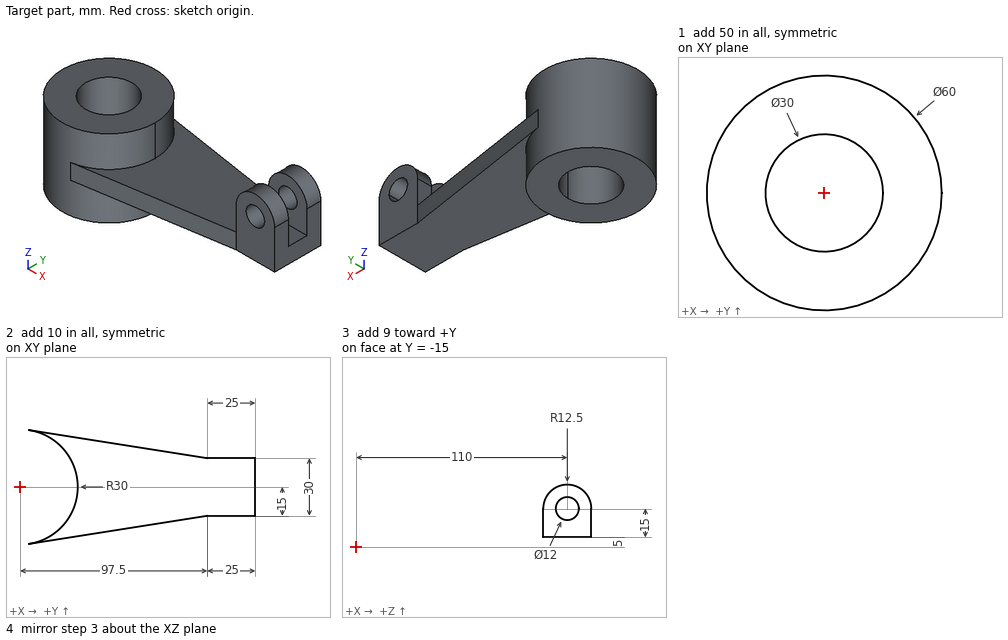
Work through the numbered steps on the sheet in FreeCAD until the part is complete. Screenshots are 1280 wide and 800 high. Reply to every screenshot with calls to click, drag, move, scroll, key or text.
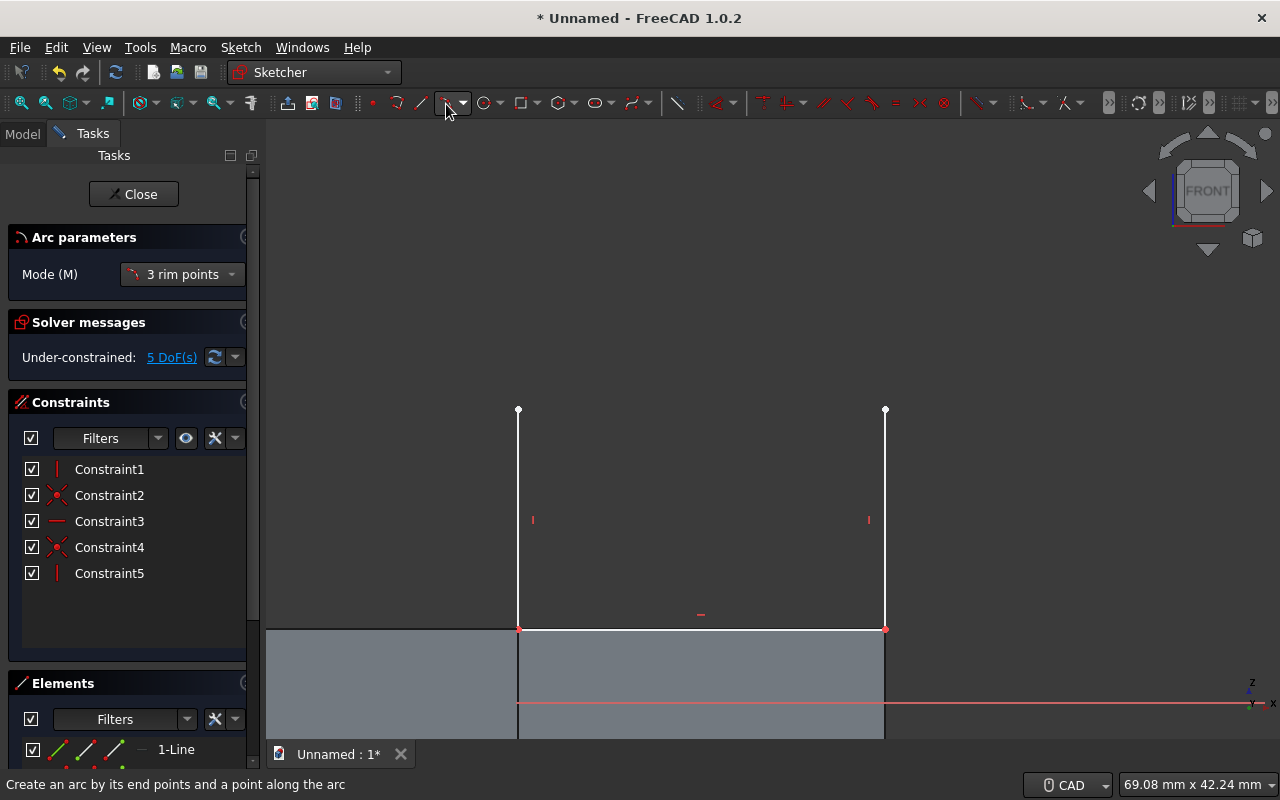
click(885, 410)
click(518, 410)
click(701, 226)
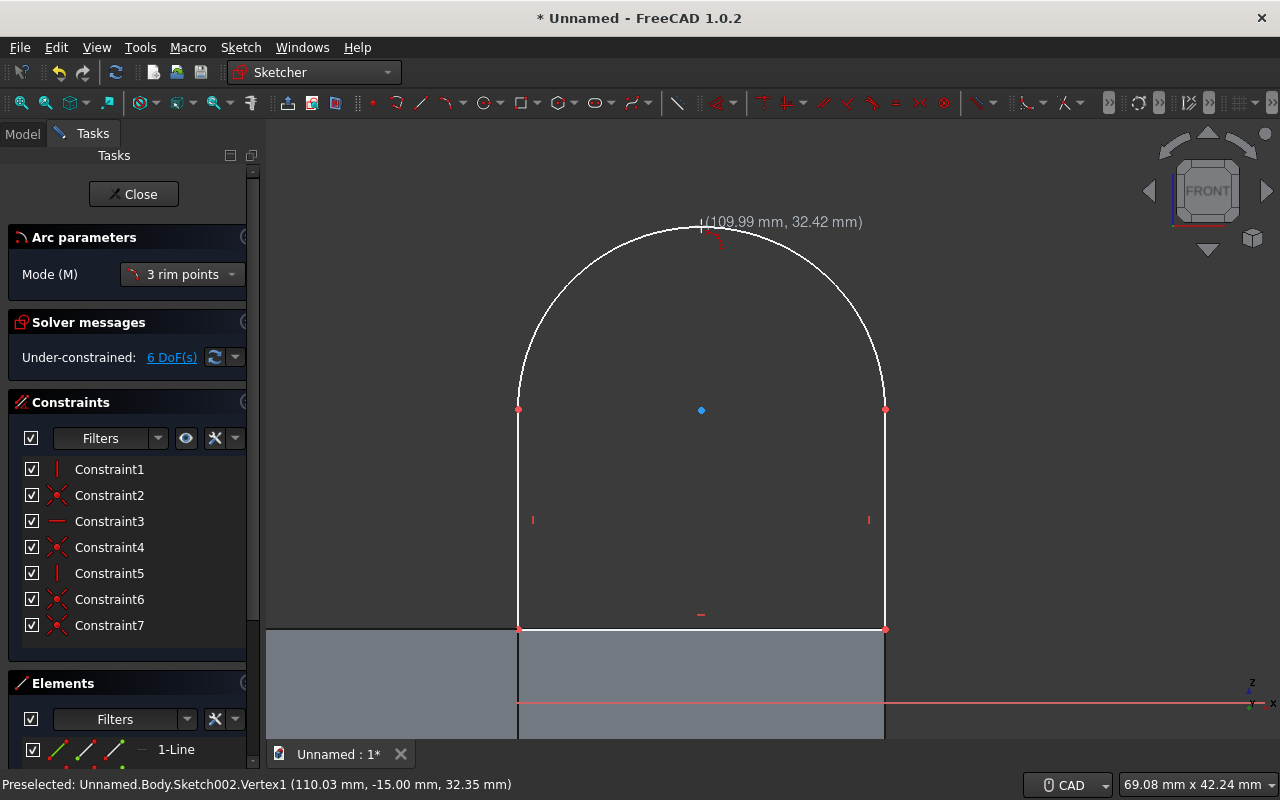
click(484, 104)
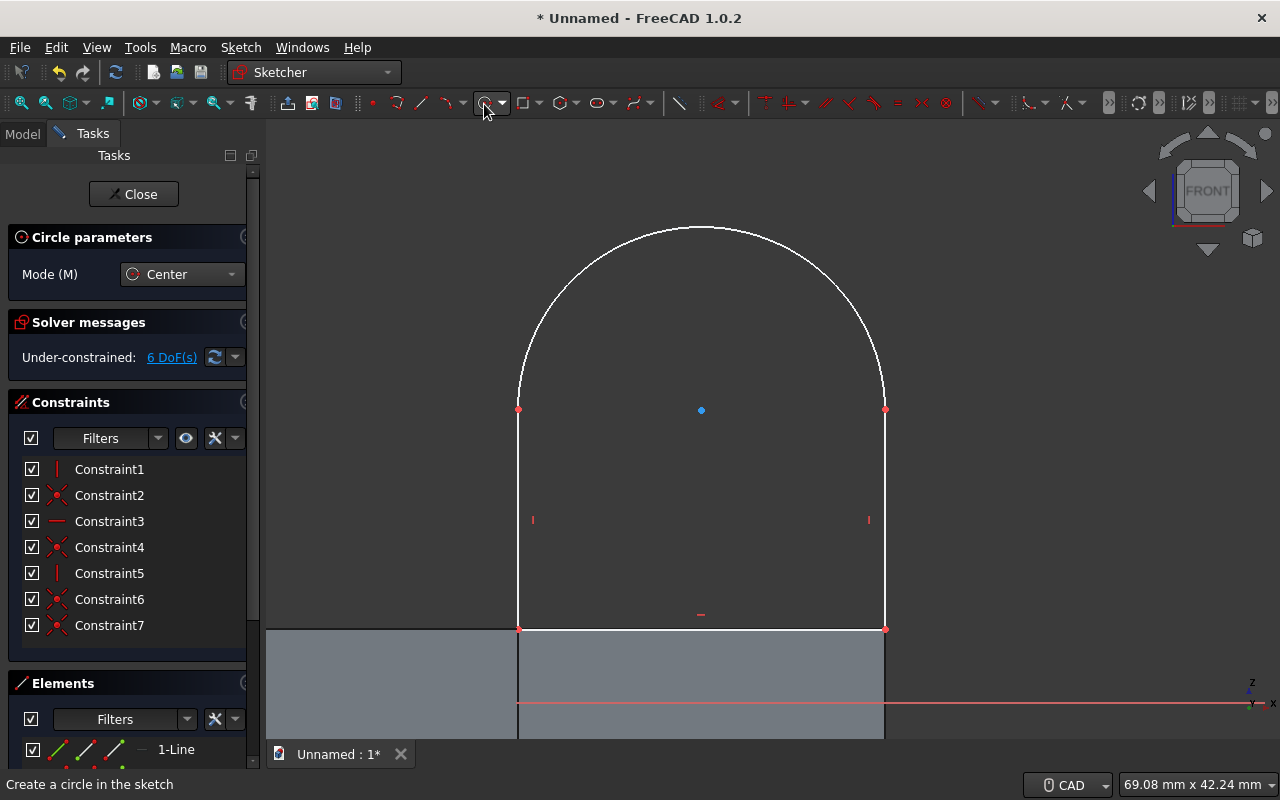
click(701, 409)
click(763, 347)
key(Escape)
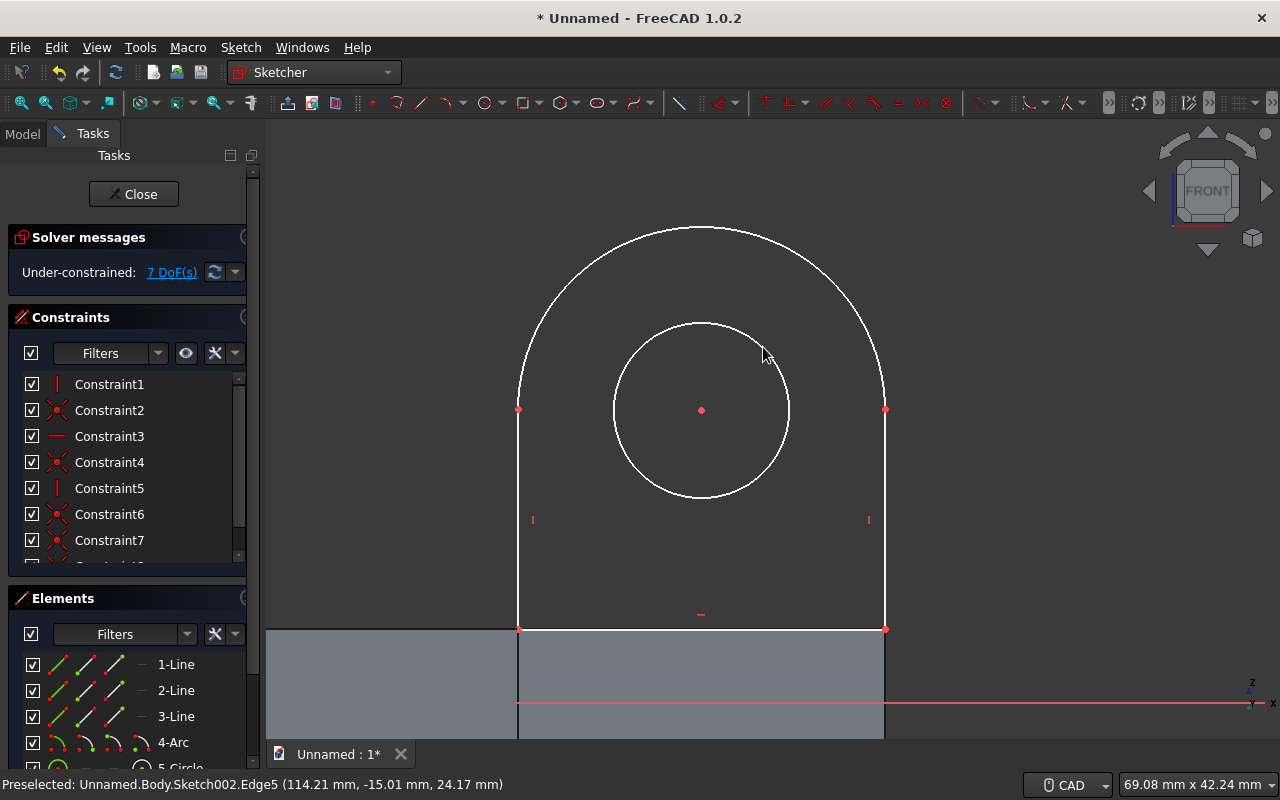
click(518, 476)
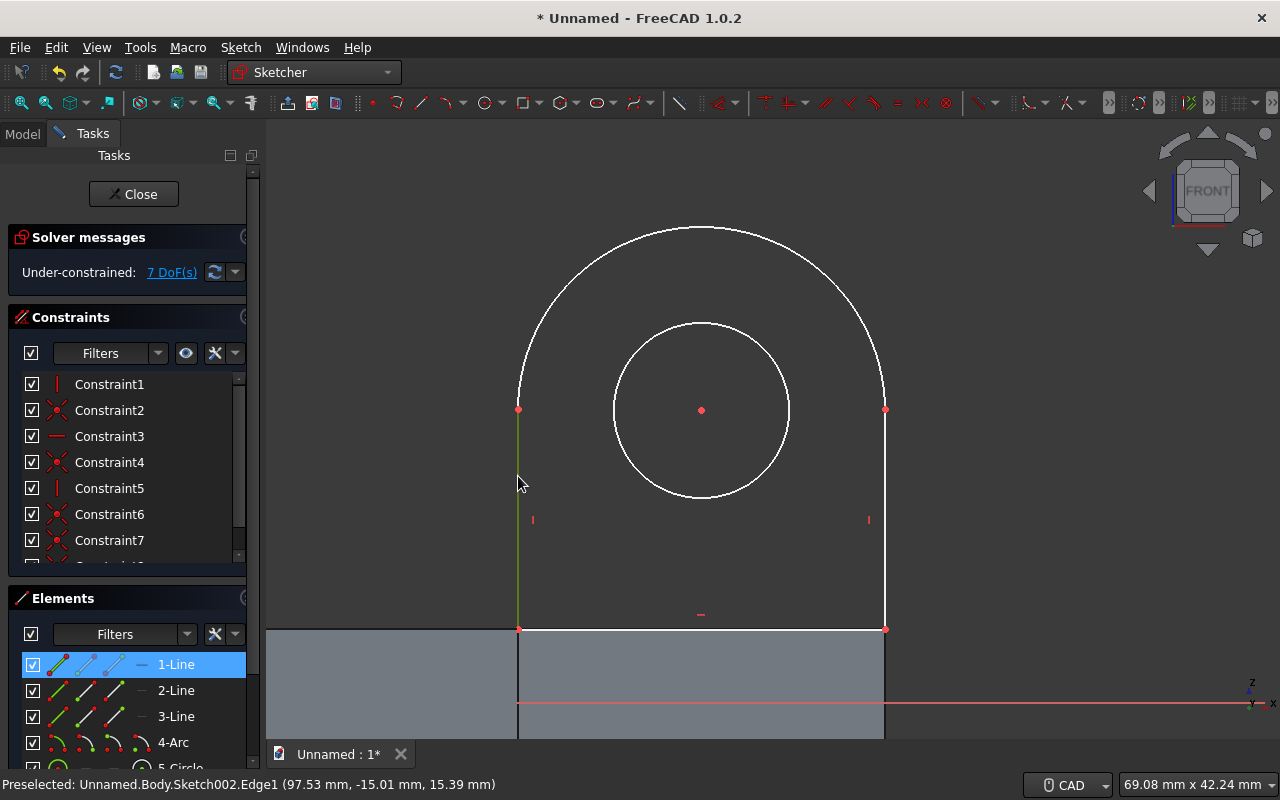
click(809, 262)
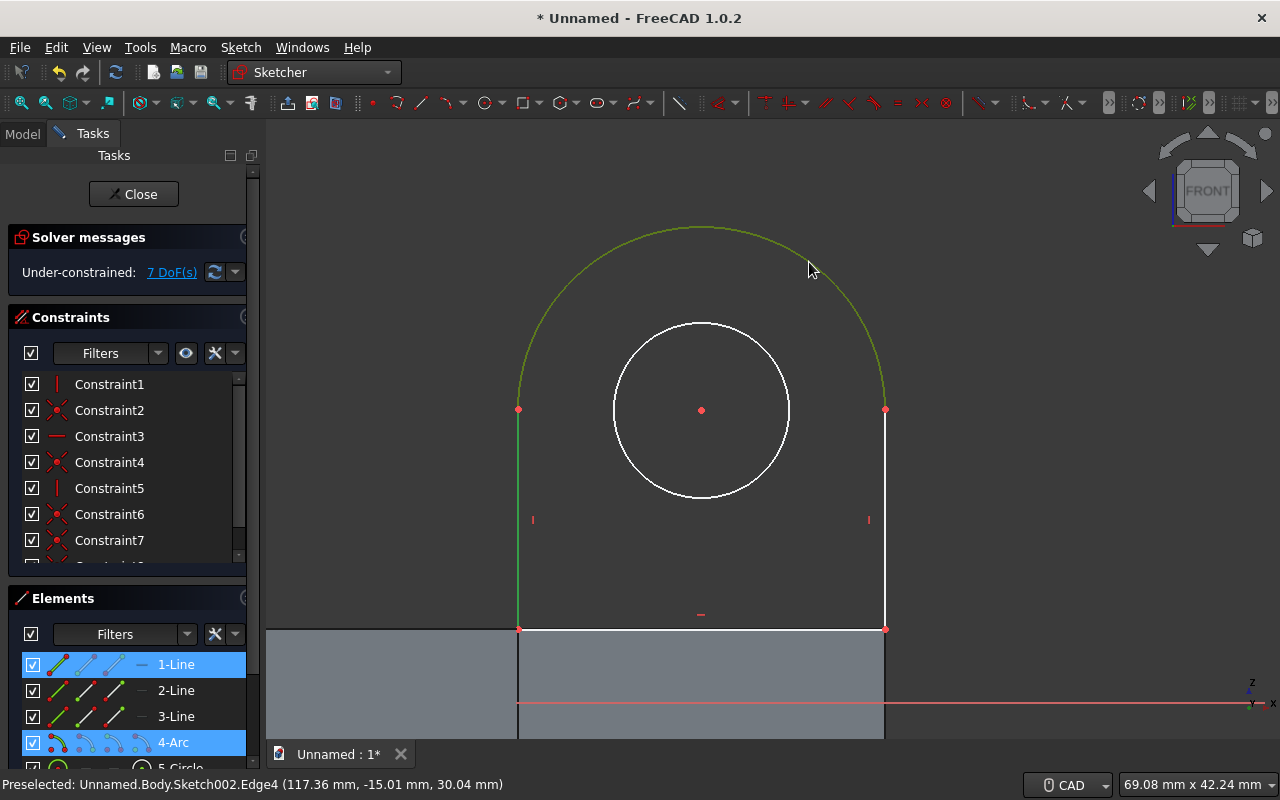
click(874, 104)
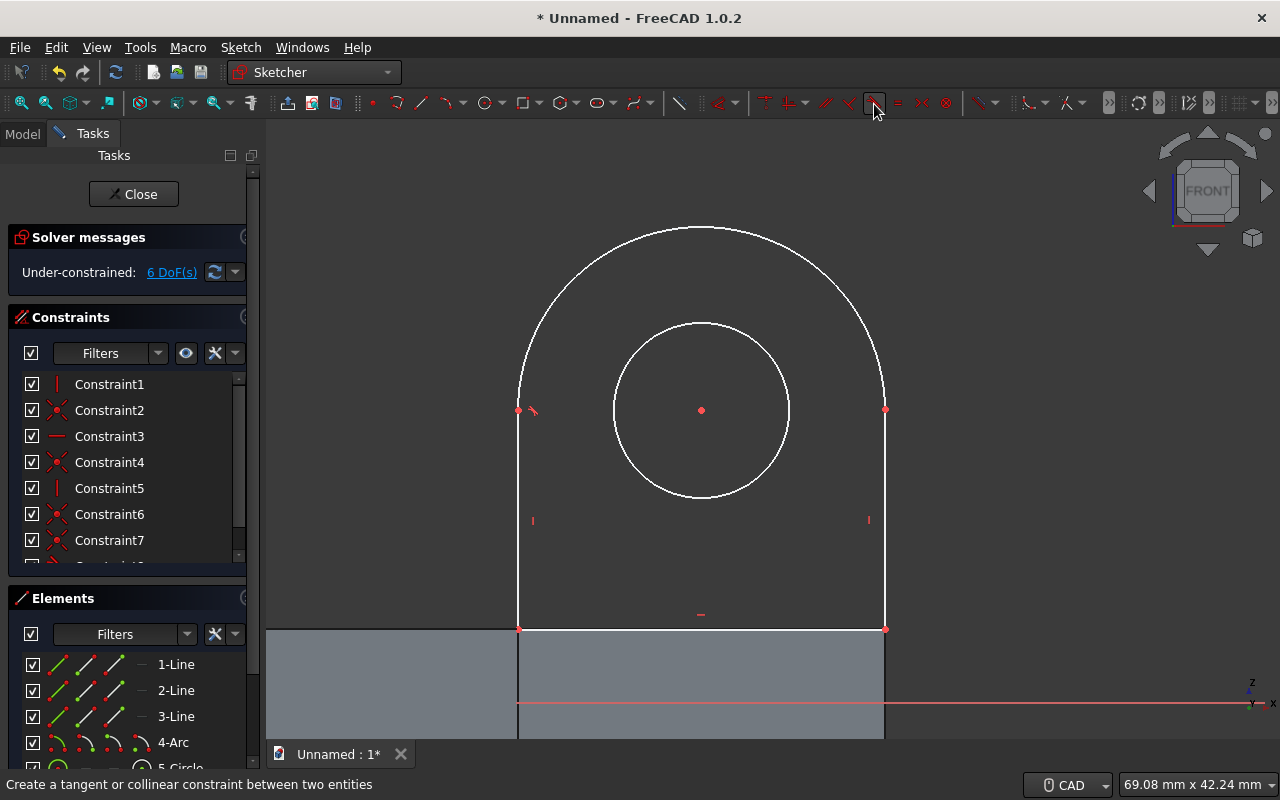
click(885, 564)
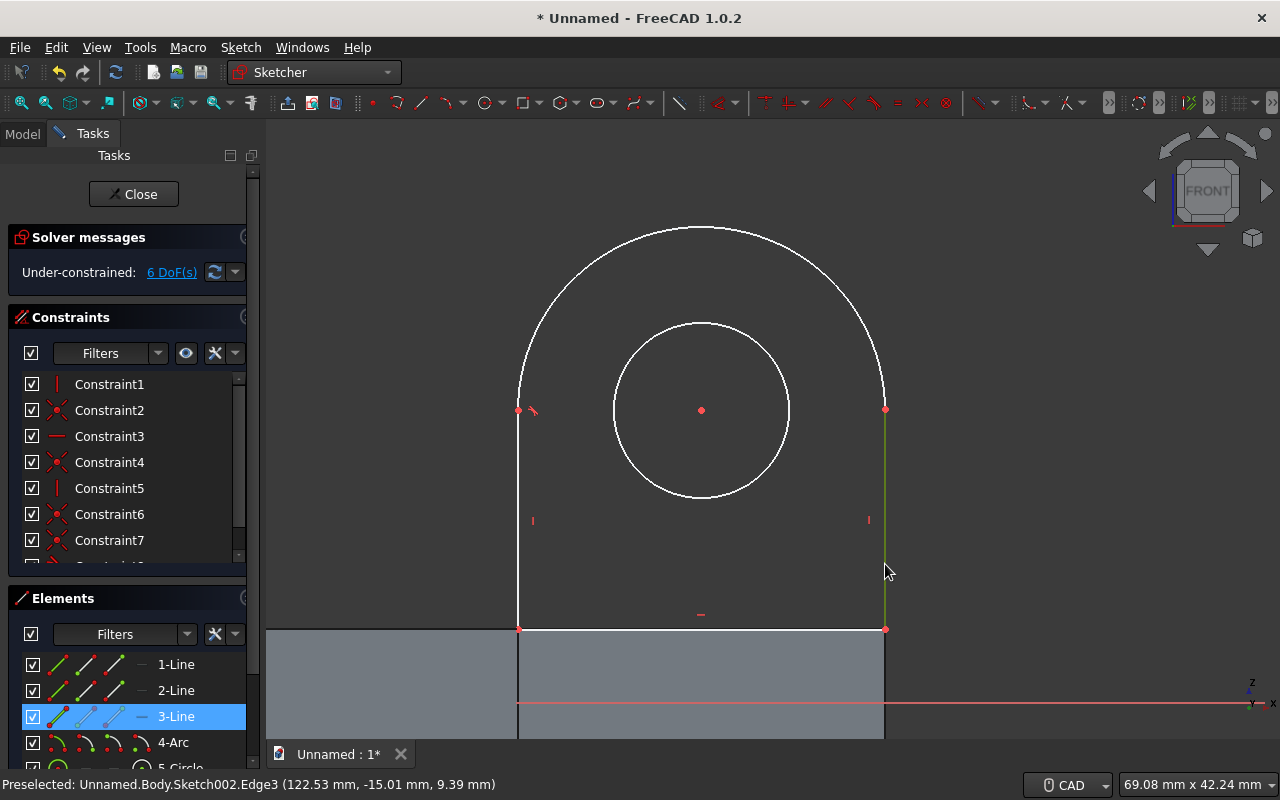
click(809, 262)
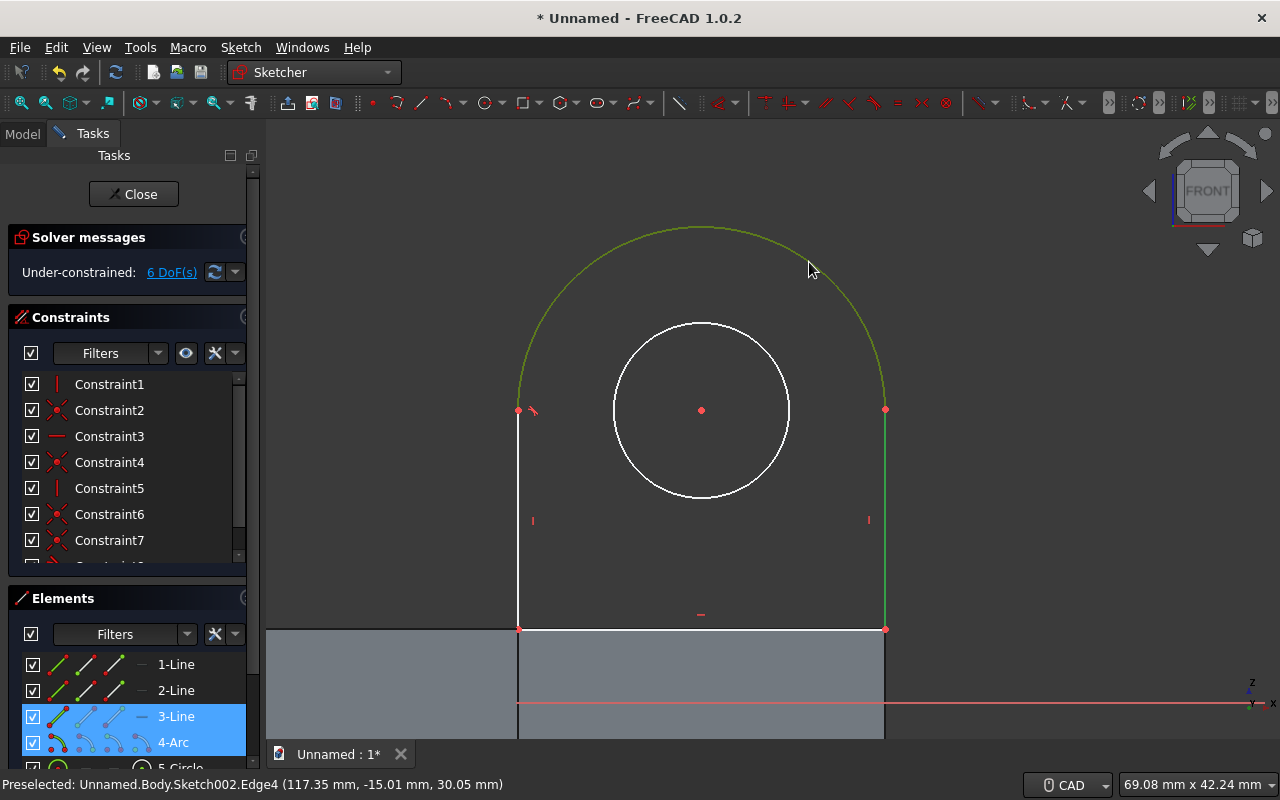
click(874, 104)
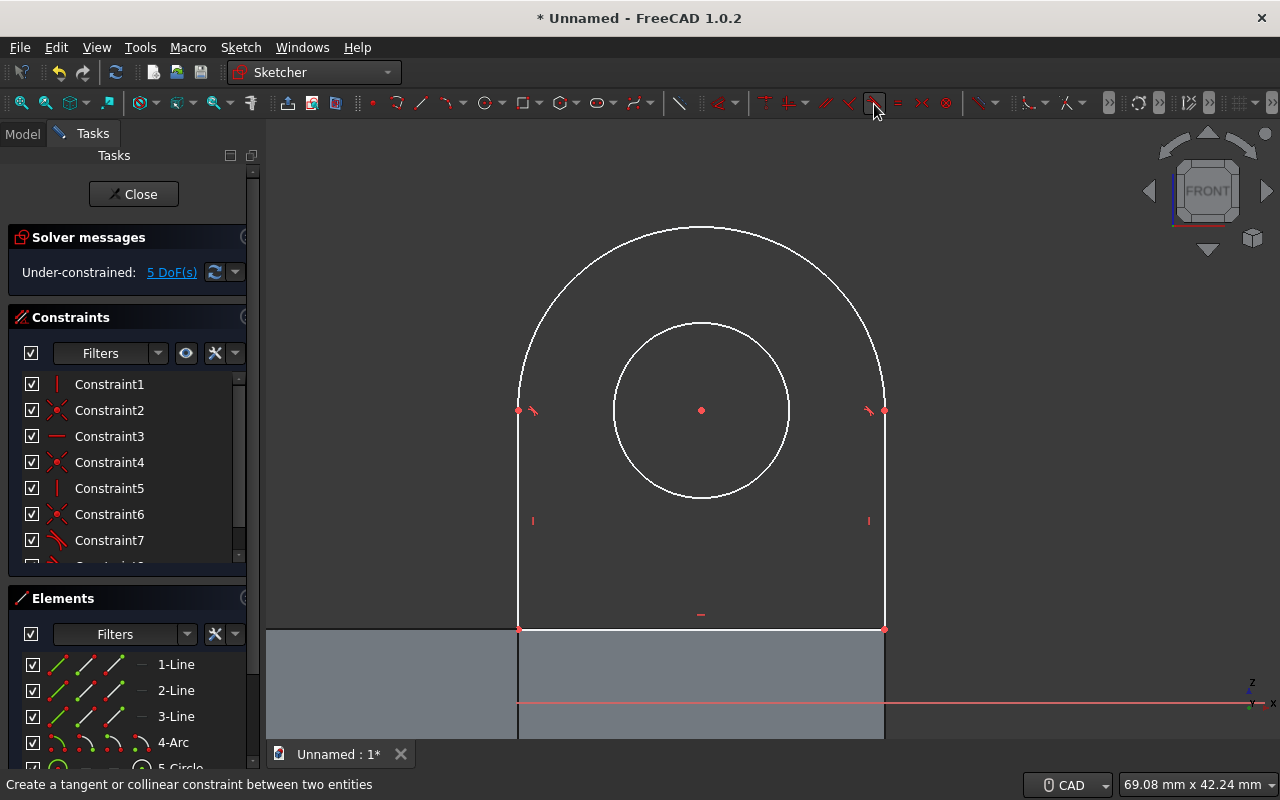
click(718, 104)